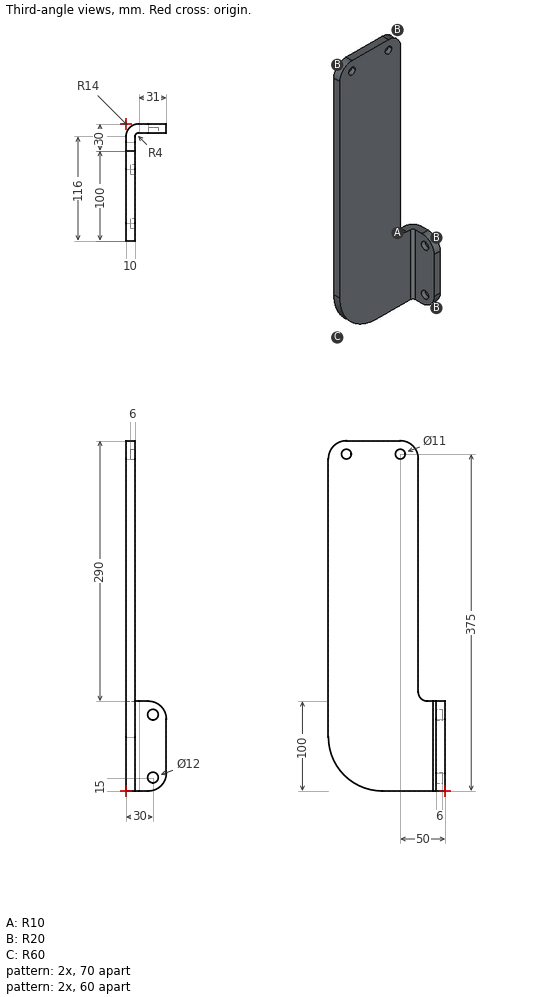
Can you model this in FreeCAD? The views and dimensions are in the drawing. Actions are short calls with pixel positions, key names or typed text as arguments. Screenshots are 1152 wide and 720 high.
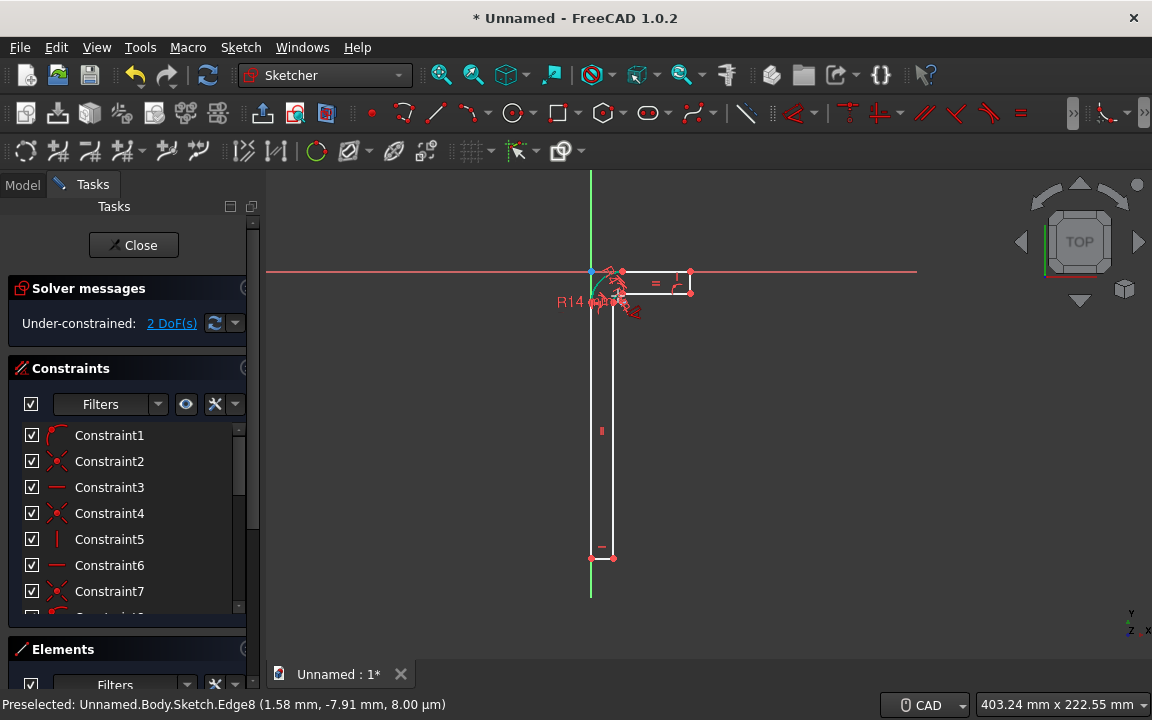
click(643, 294)
click(656, 328)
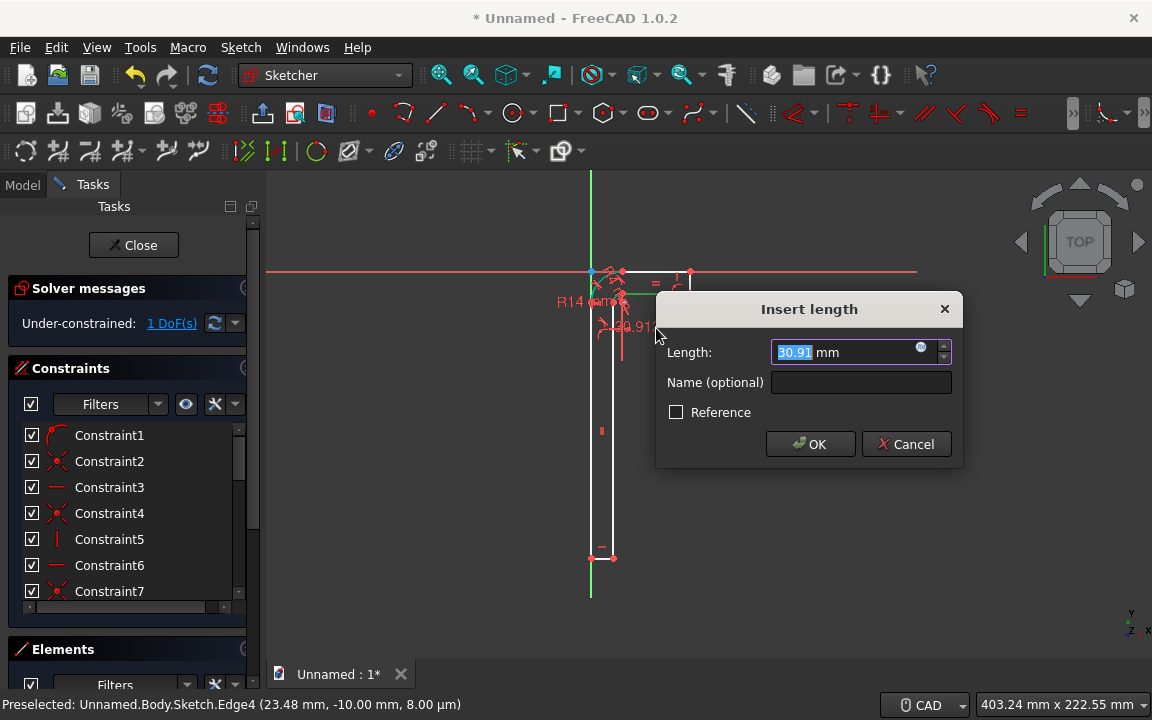
text(31)
key(Return)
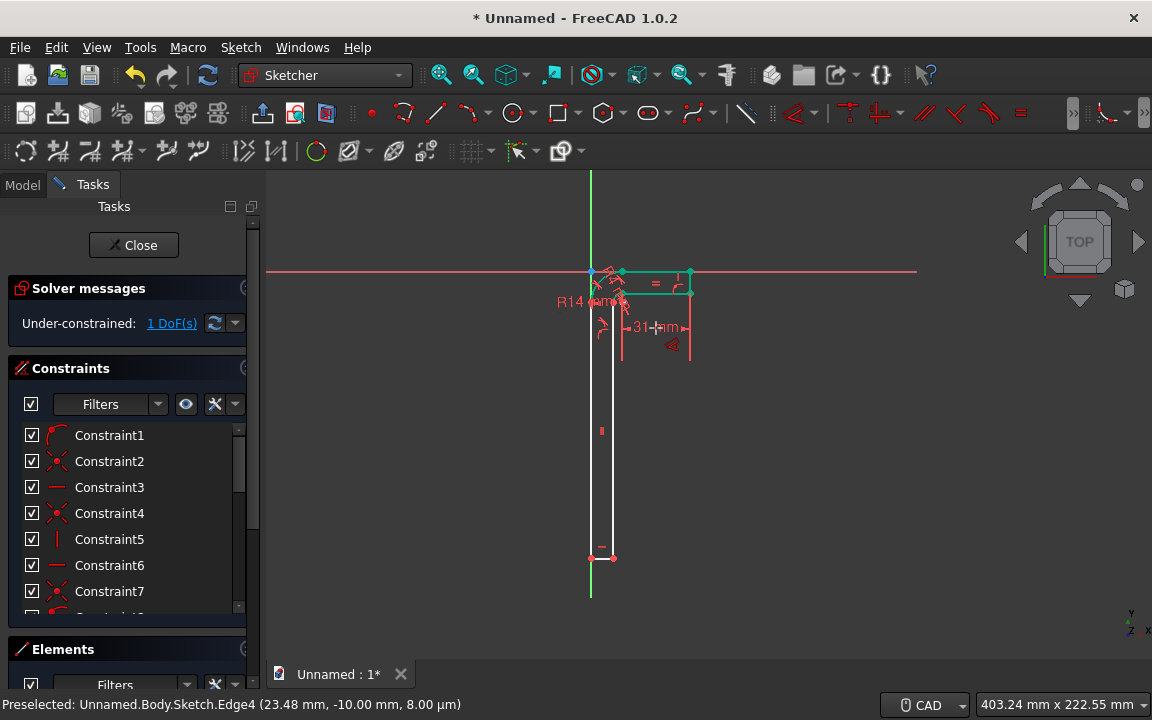
click(591, 379)
click(557, 431)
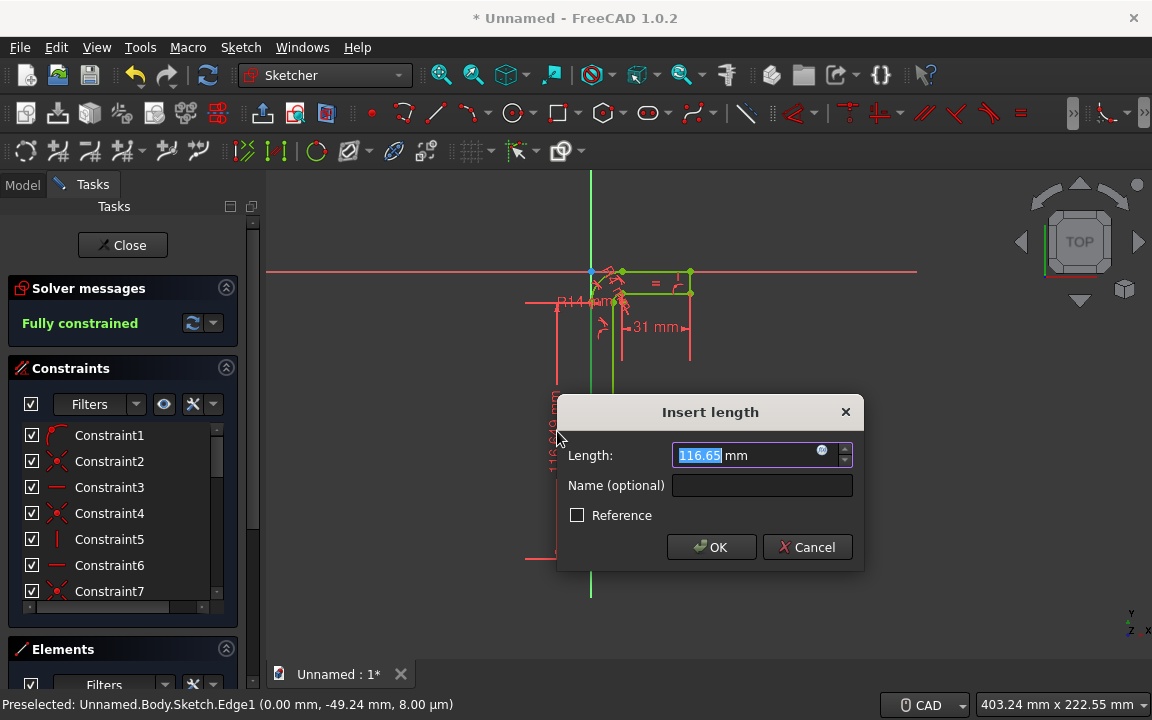
text(116)
key(Return)
key(Escape)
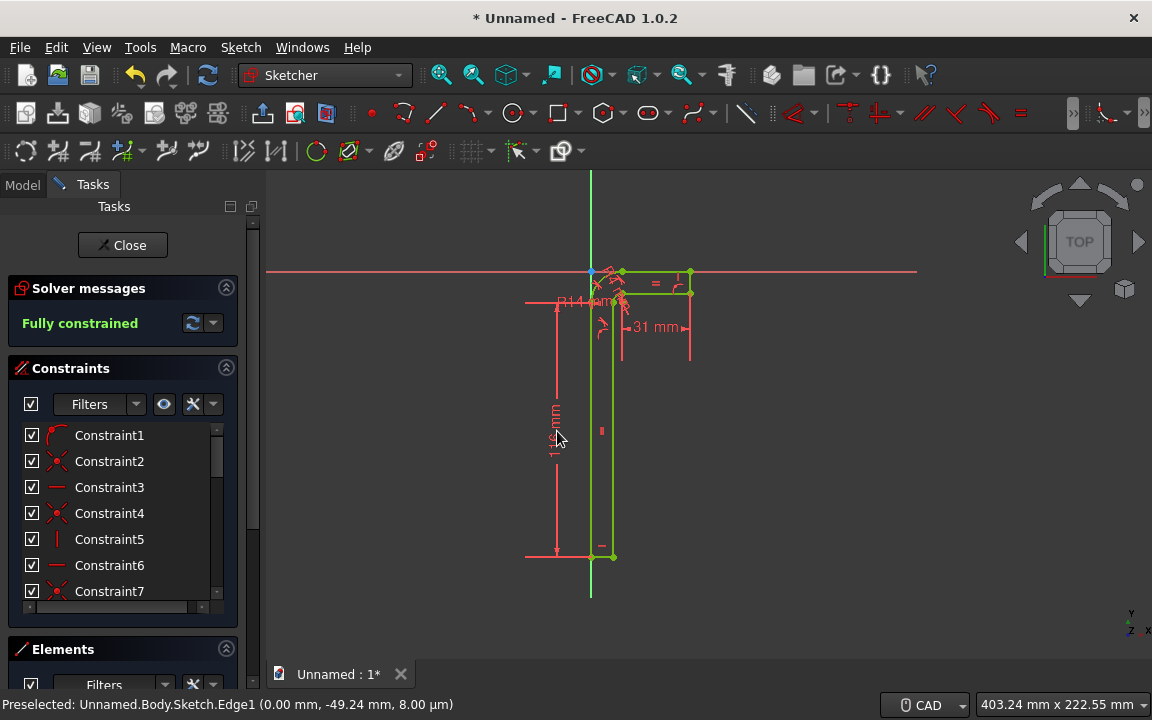
click(123, 245)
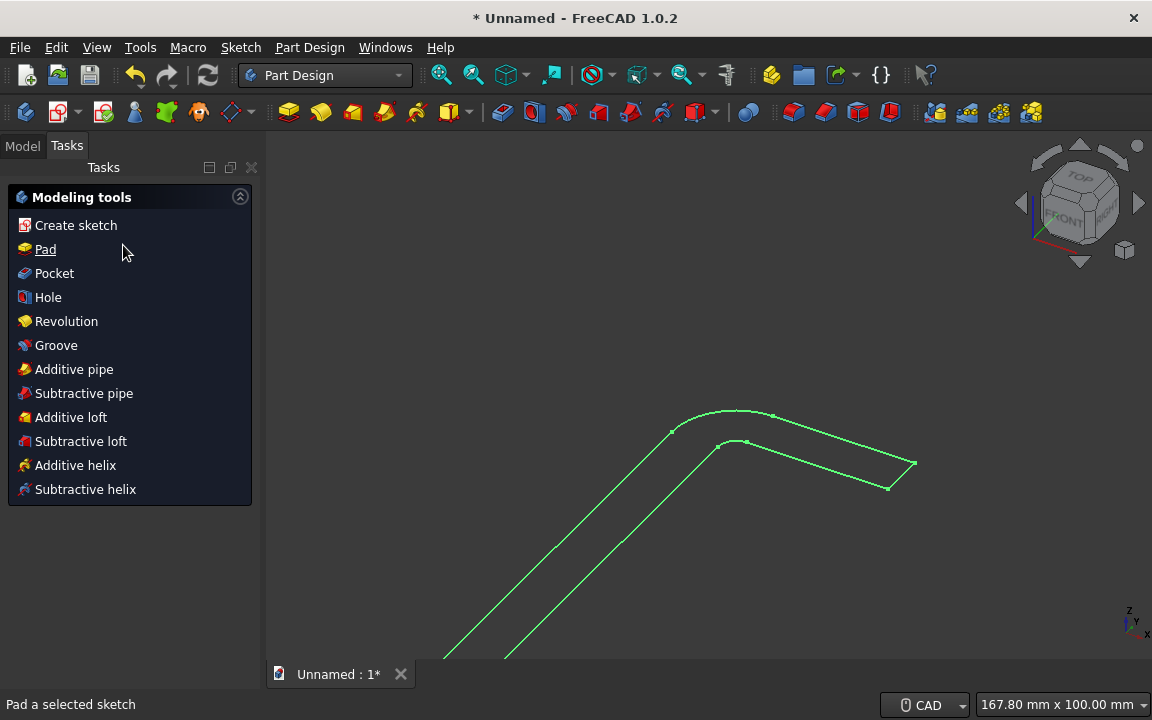
click(290, 112)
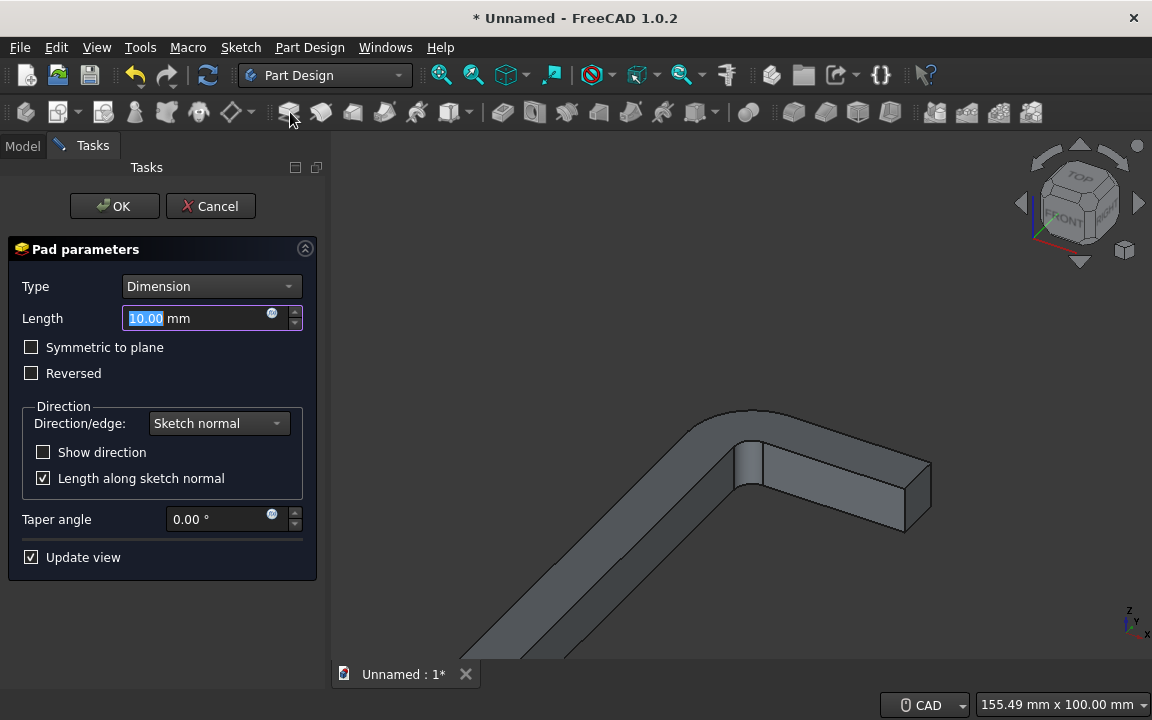
text(100)
key(Tab)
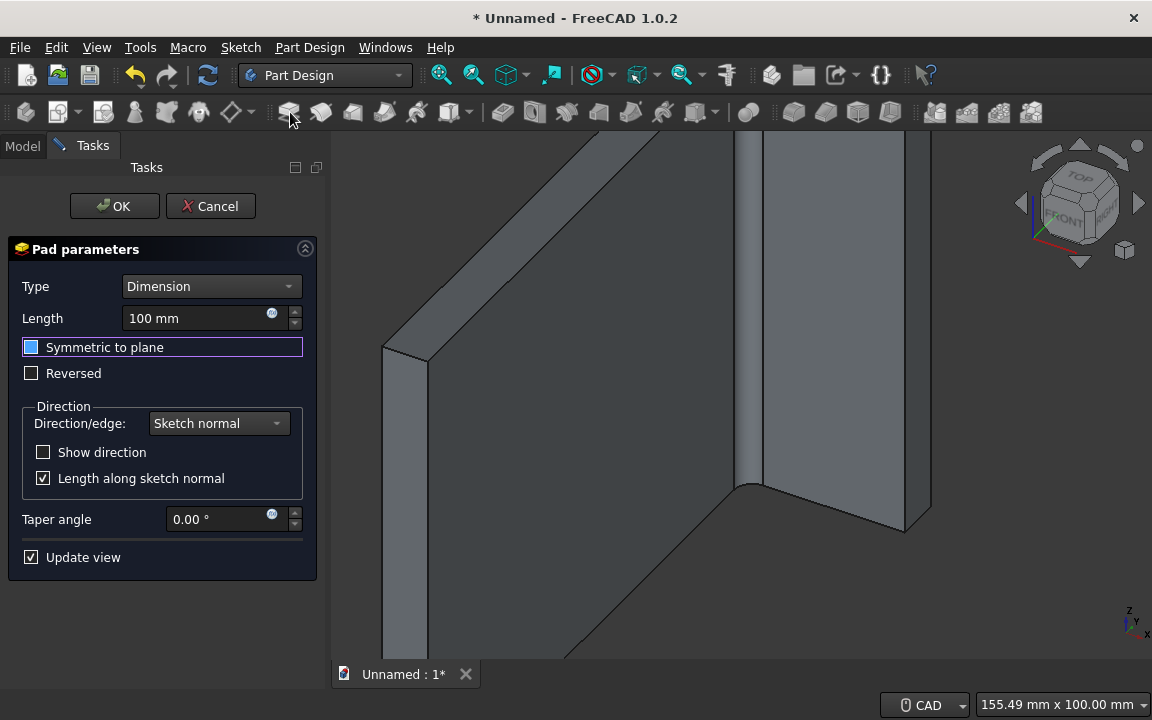
click(115, 206)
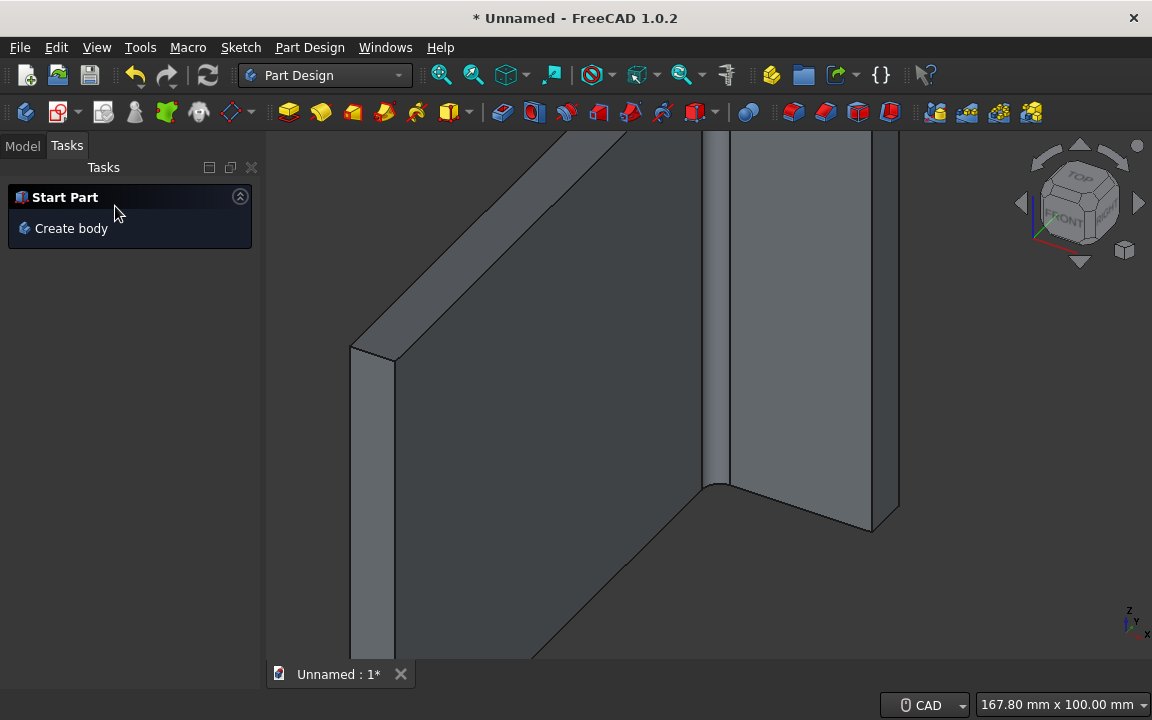
click(442, 76)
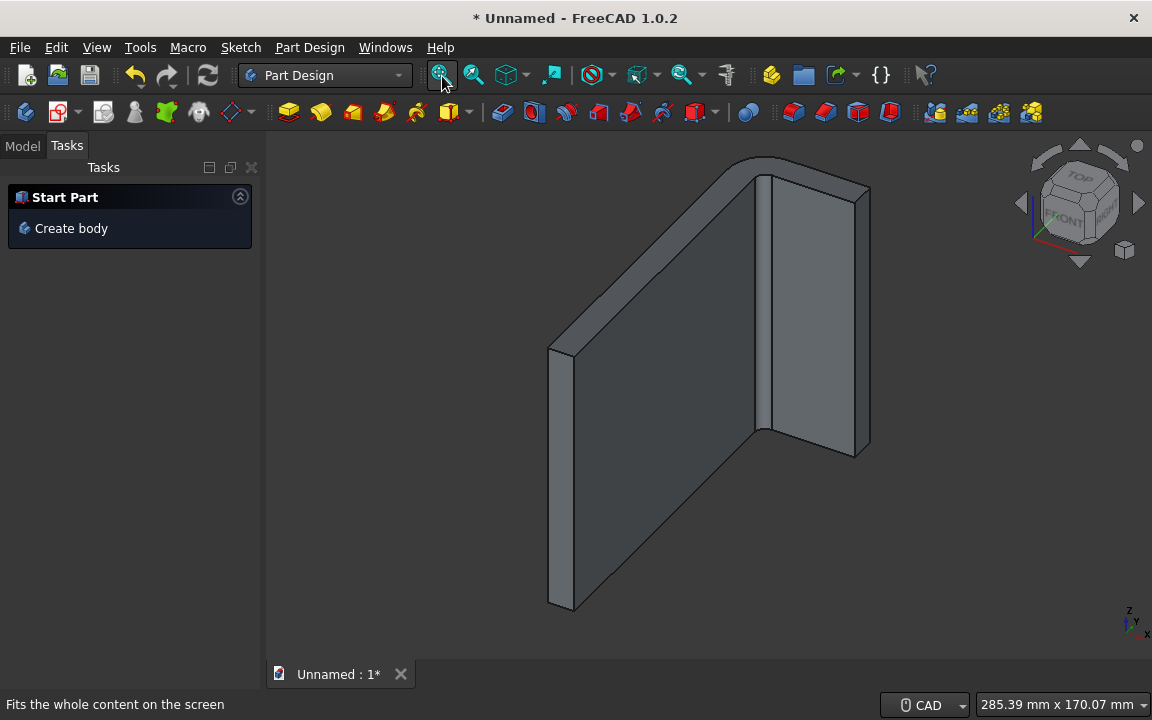
click(715, 192)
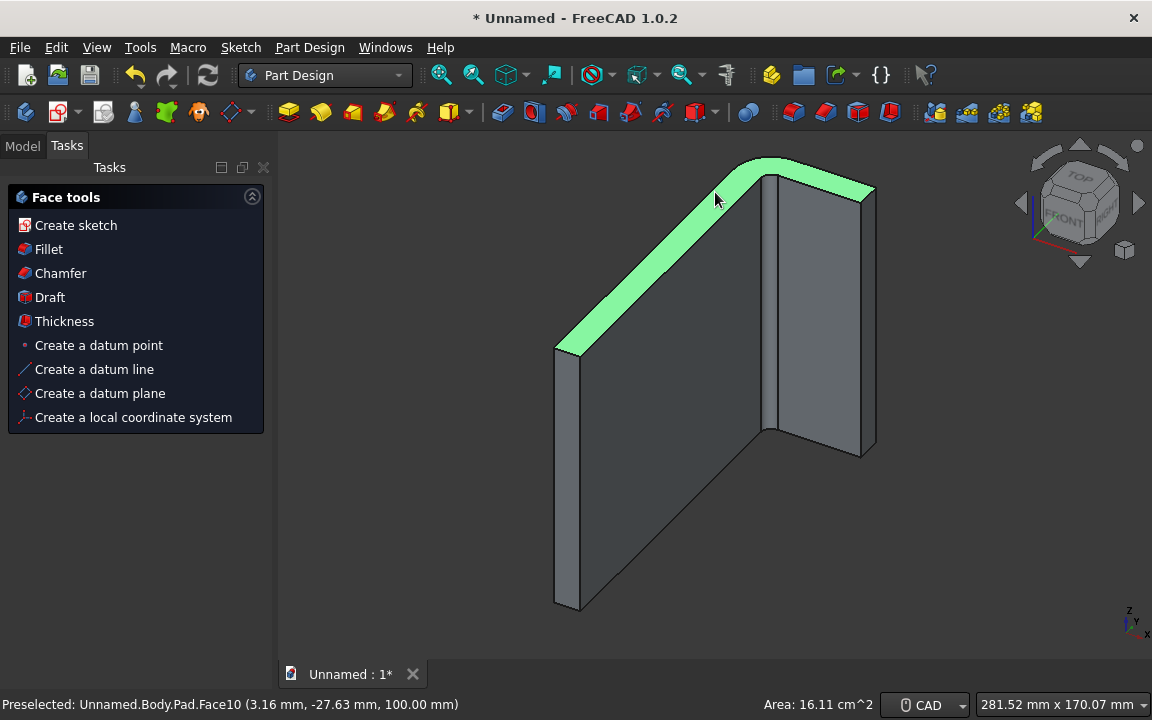
click(58, 112)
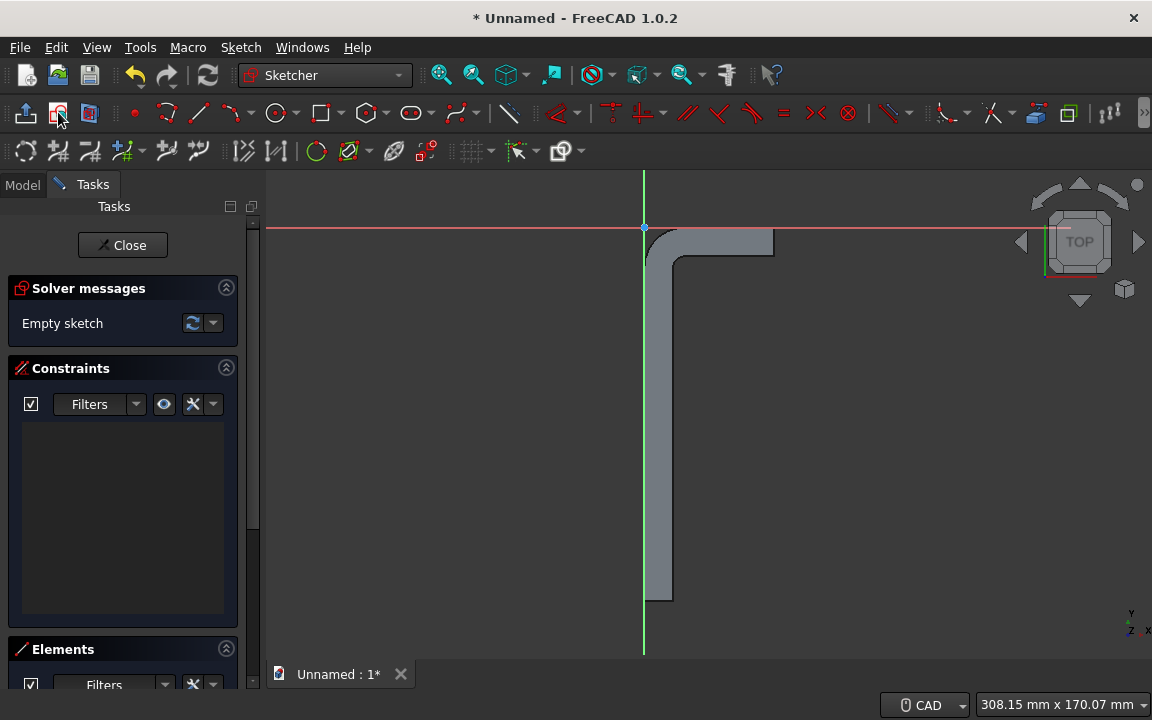
click(322, 114)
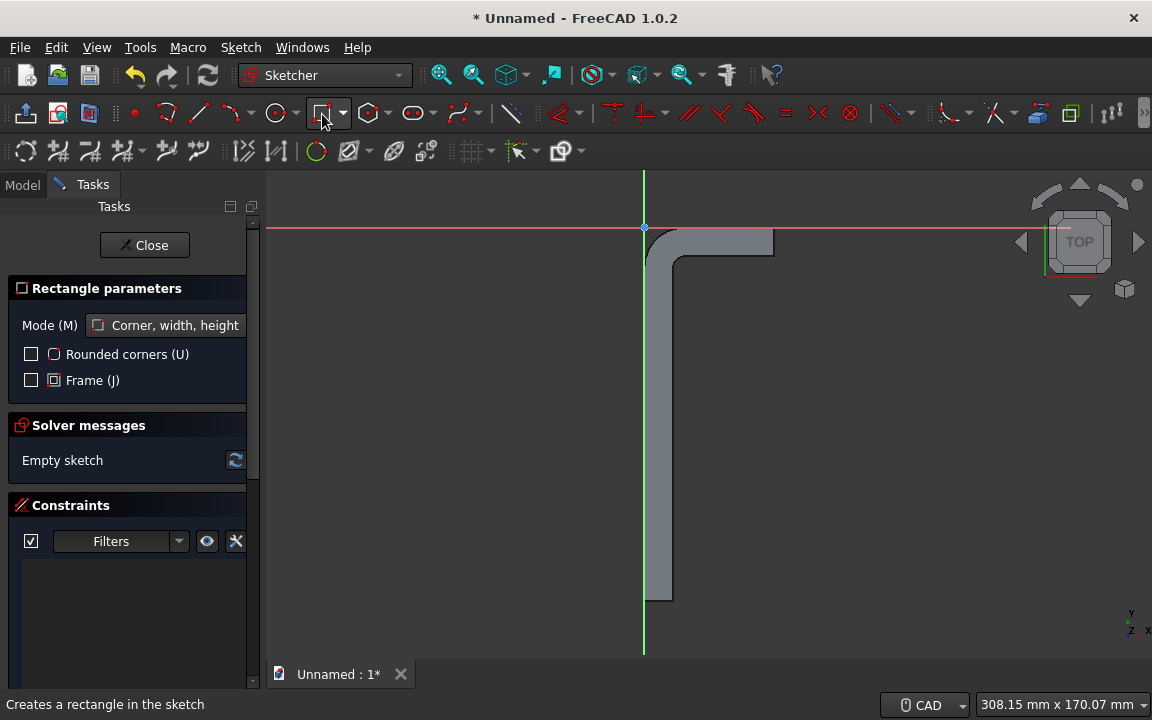
click(644, 314)
move(673, 601)